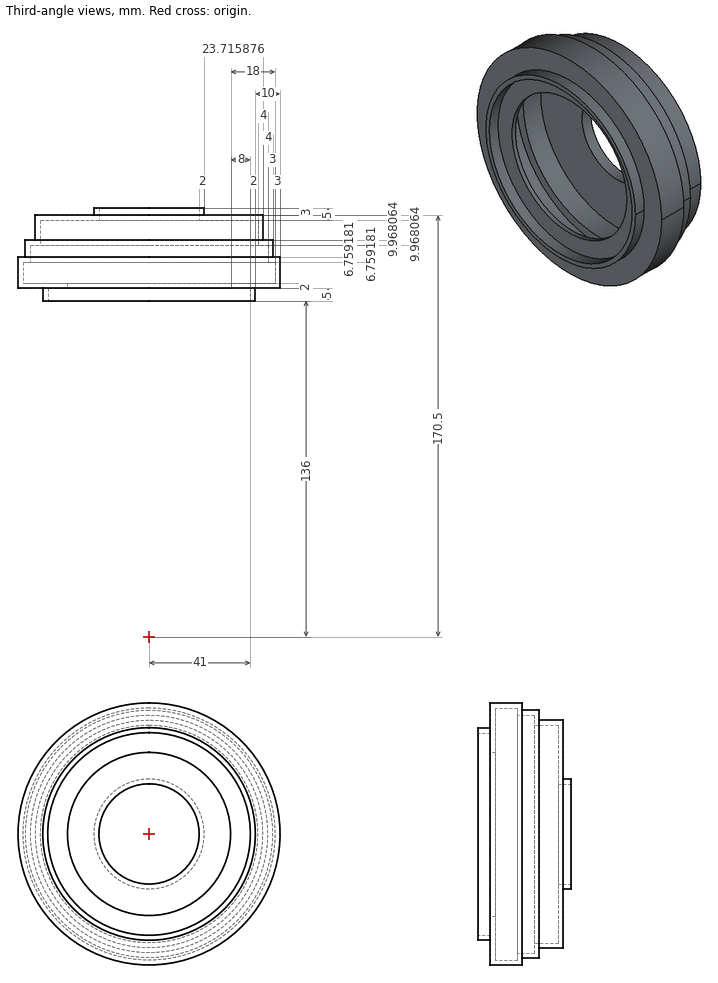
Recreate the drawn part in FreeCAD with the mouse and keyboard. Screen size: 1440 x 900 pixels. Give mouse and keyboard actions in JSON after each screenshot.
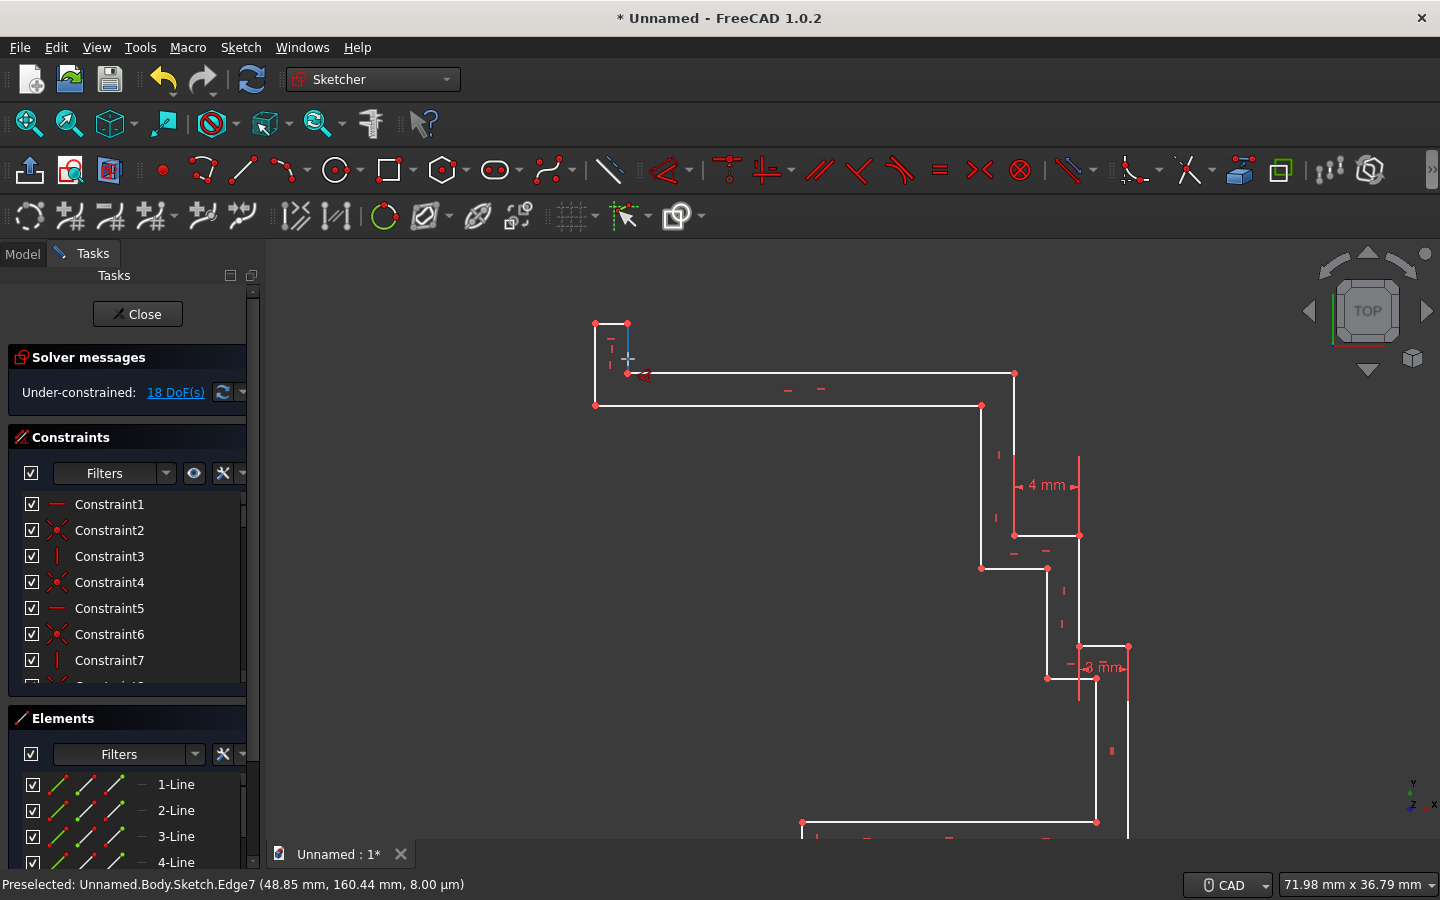
{"action": "left_click", "coordinate": [628, 358]}
{"action": "left_click", "coordinate": [662, 348]}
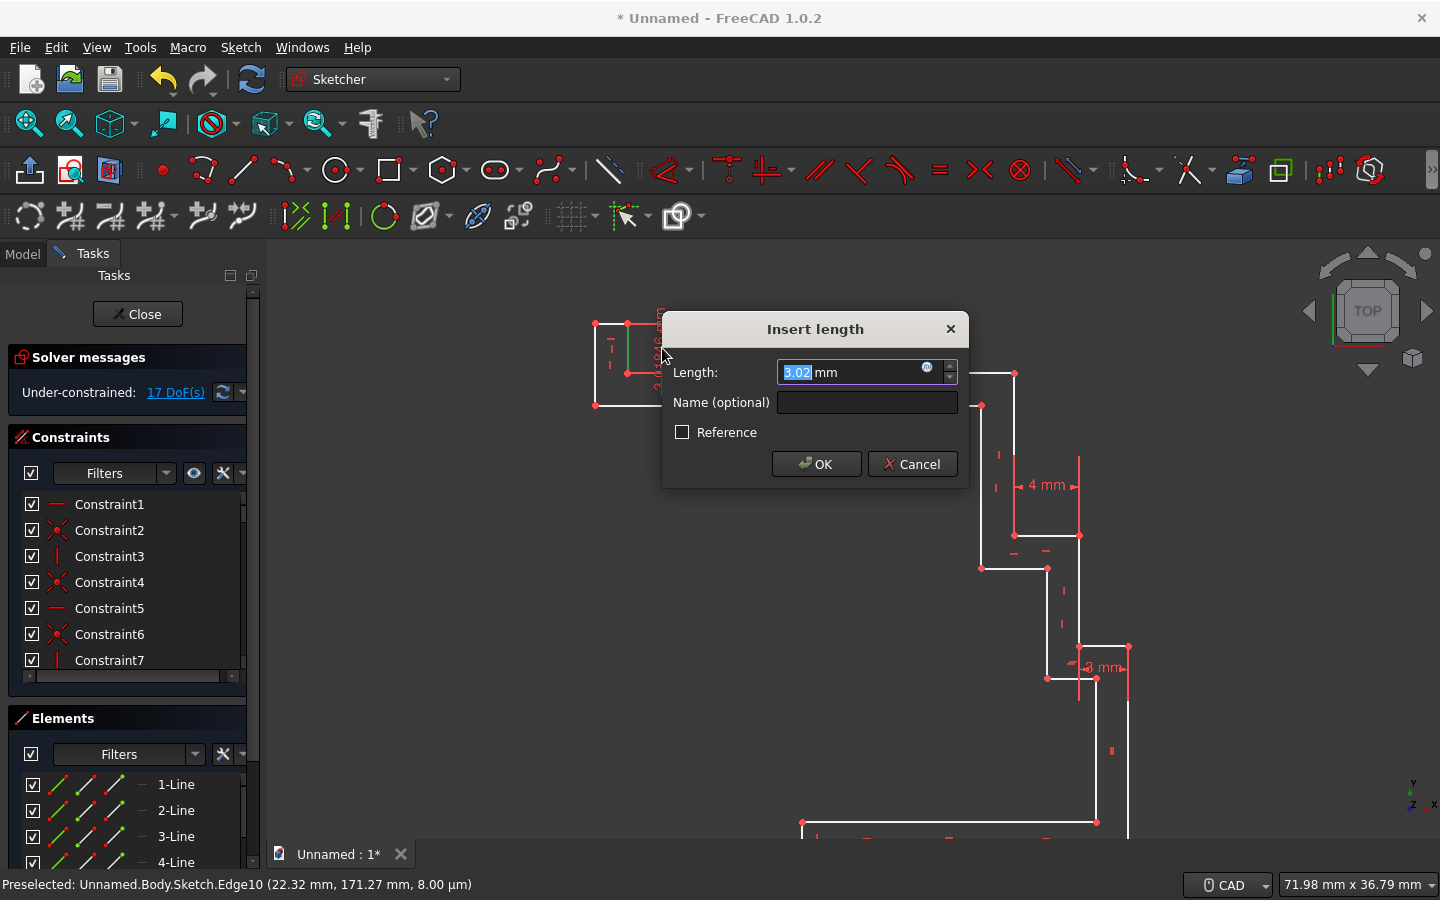
{"action": "type", "text": "3"}
{"action": "key", "text": "Return"}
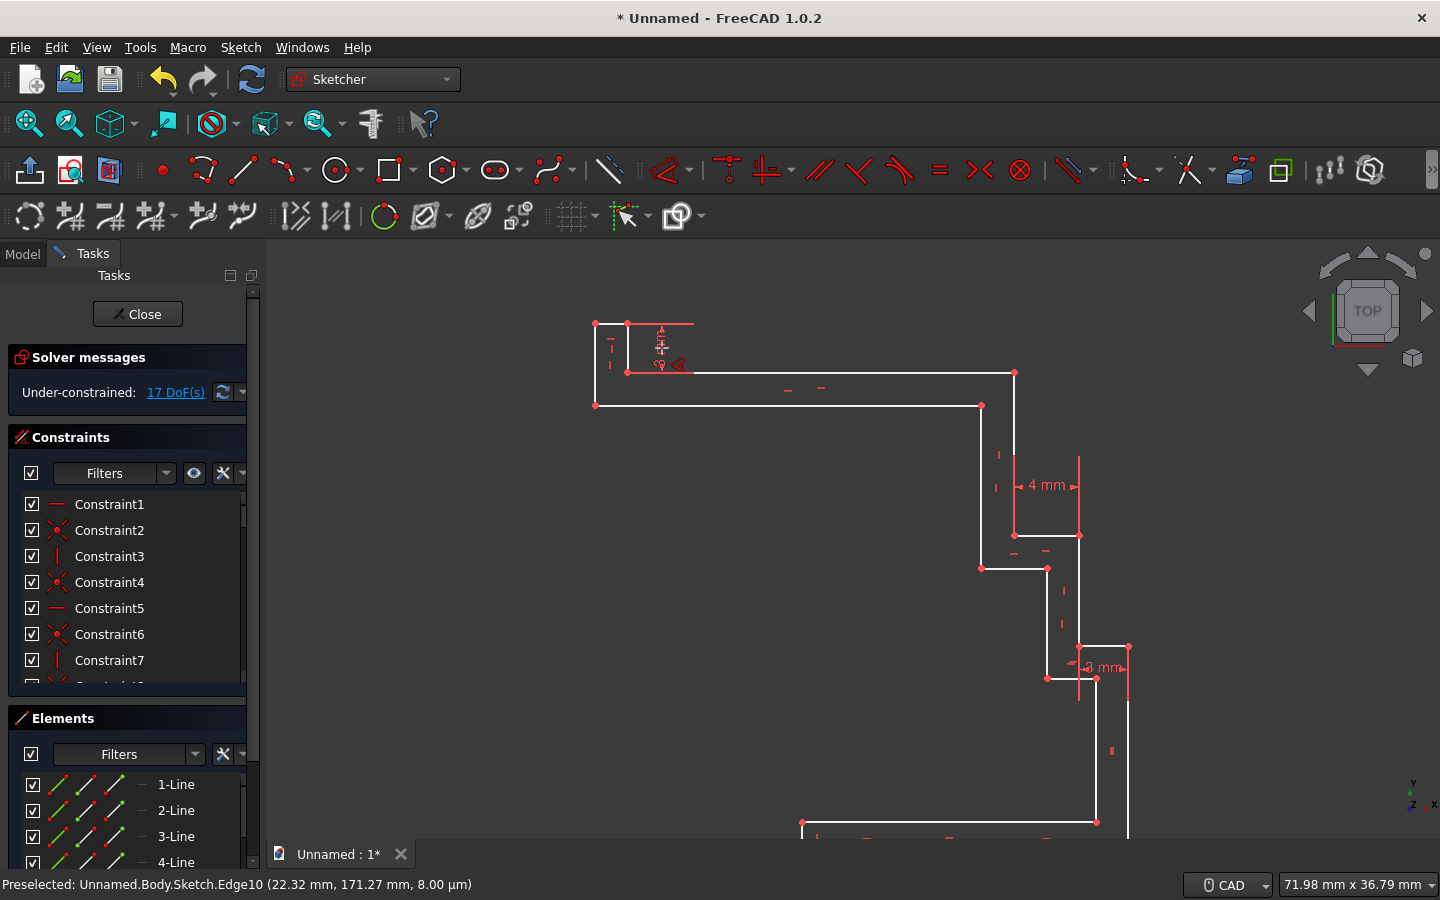
{"action": "scroll", "coordinate": [618, 324], "scroll_direction": "up", "scroll_amount": 2}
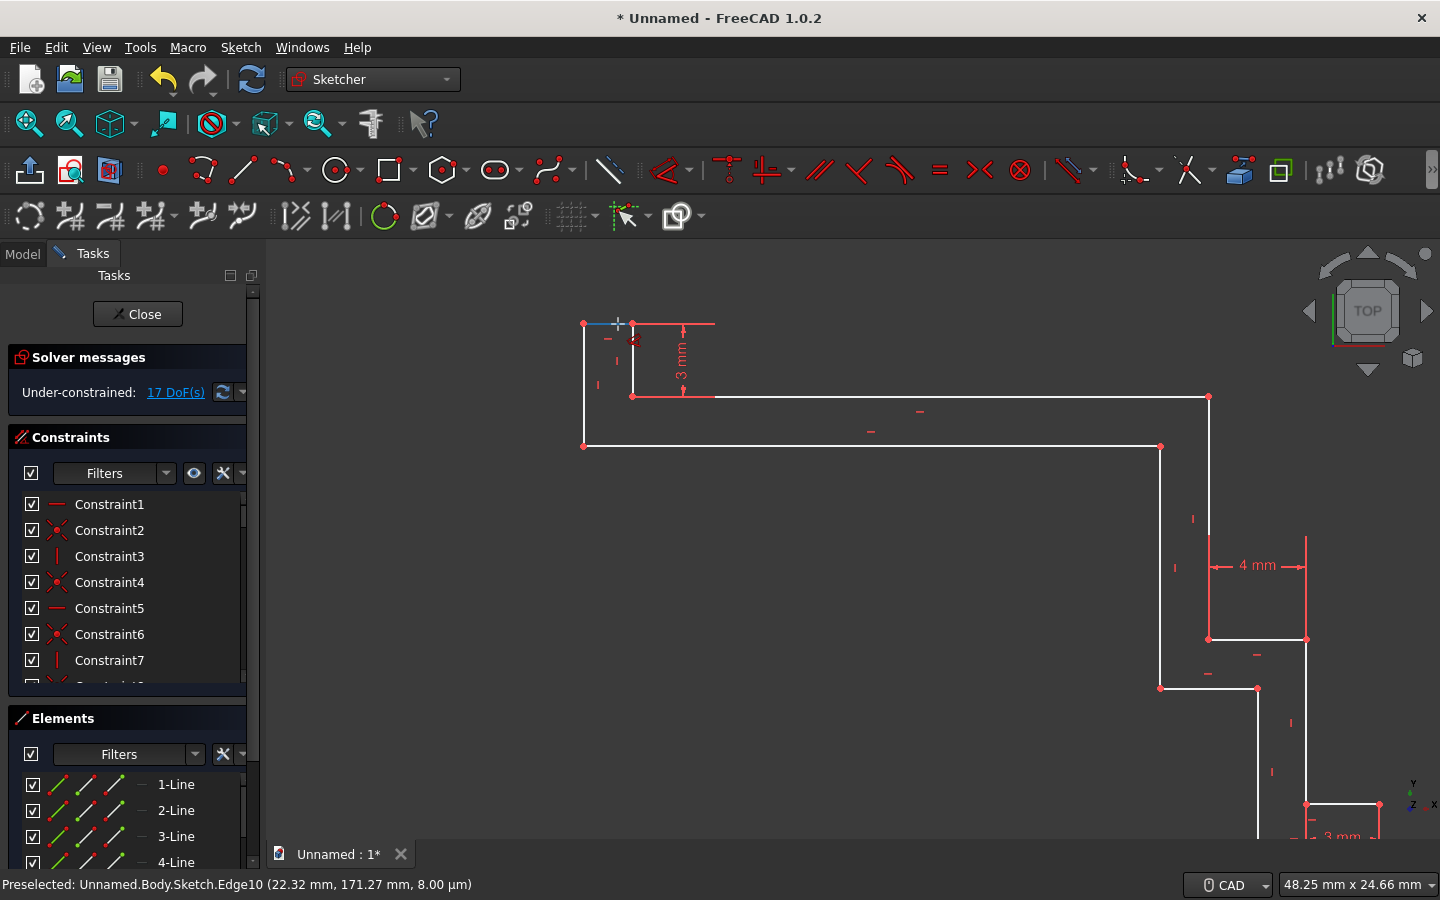
{"action": "left_click", "coordinate": [618, 324]}
{"action": "left_click", "coordinate": [608, 290]}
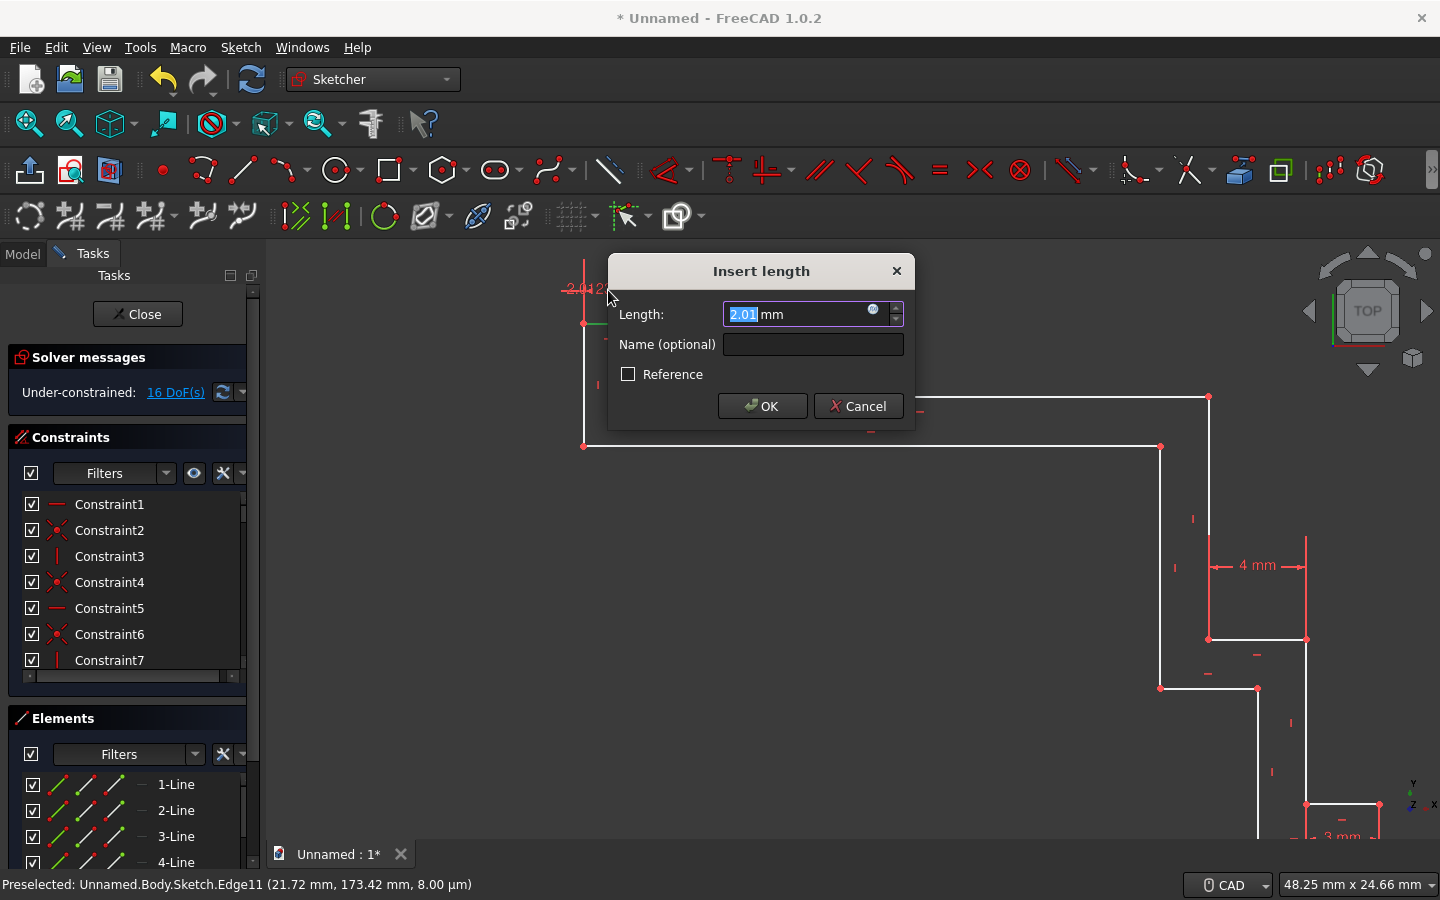
{"action": "type", "text": "2"}
{"action": "key", "text": "Return"}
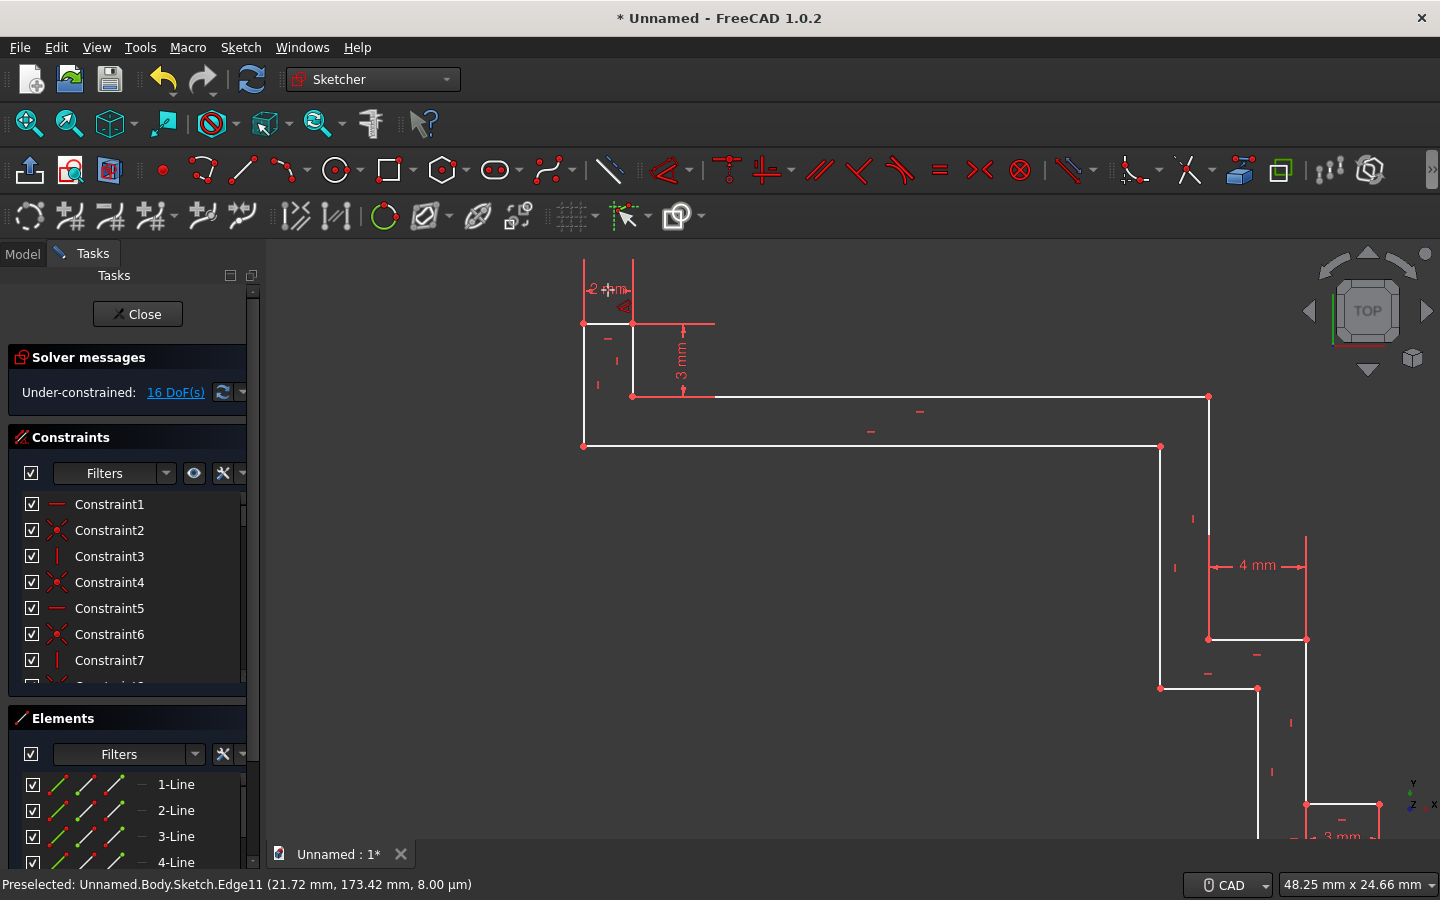
{"action": "left_click", "coordinate": [584, 360]}
{"action": "left_click", "coordinate": [550, 385]}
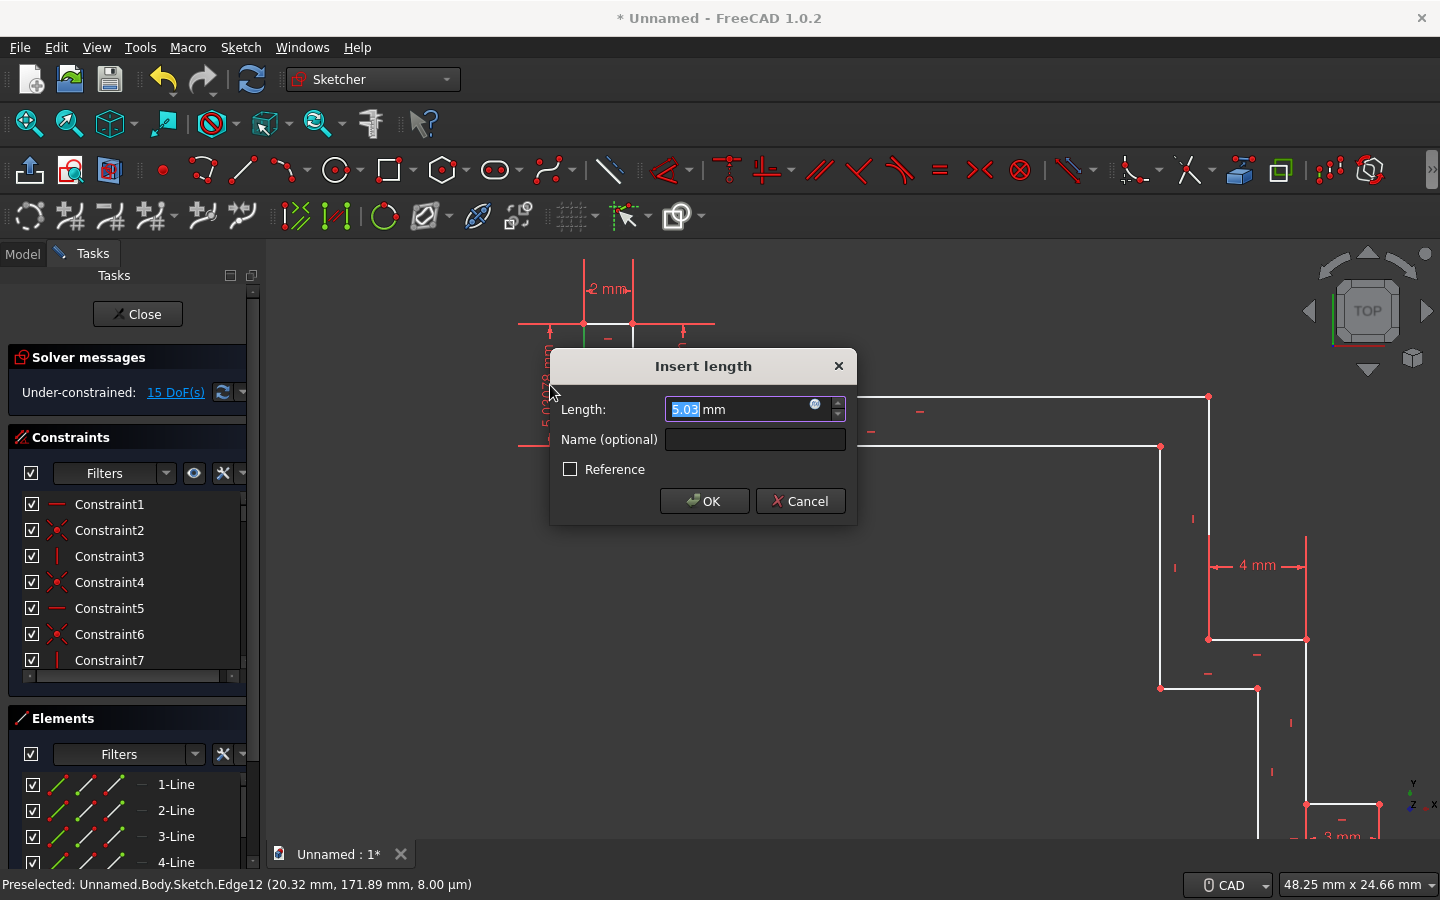
{"action": "type", "text": "5"}
{"action": "key", "text": "Return"}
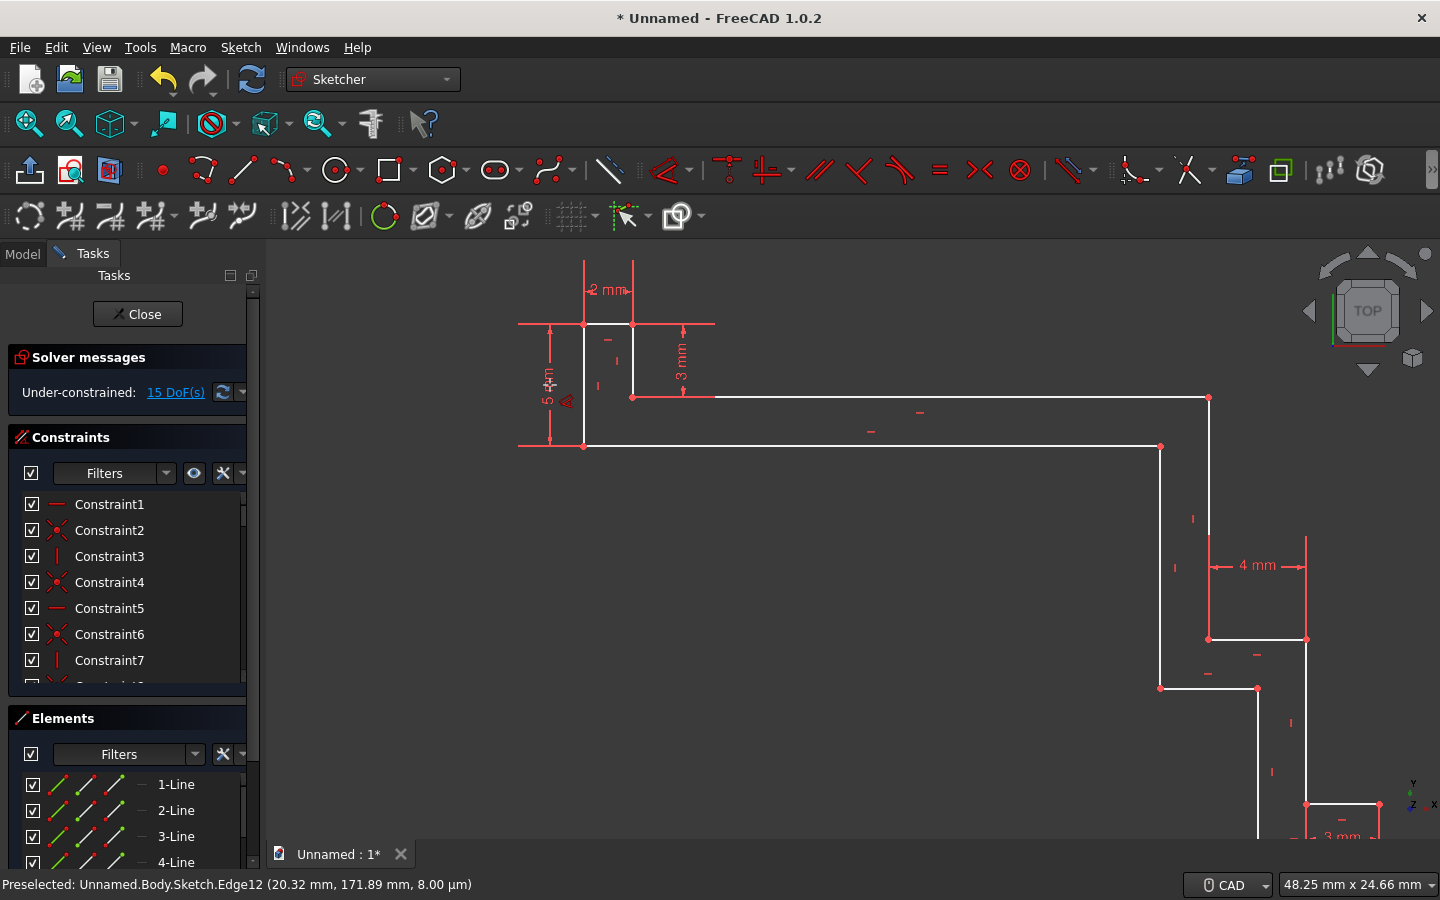
{"action": "left_click", "coordinate": [1189, 689]}
{"action": "left_click", "coordinate": [1209, 655]}